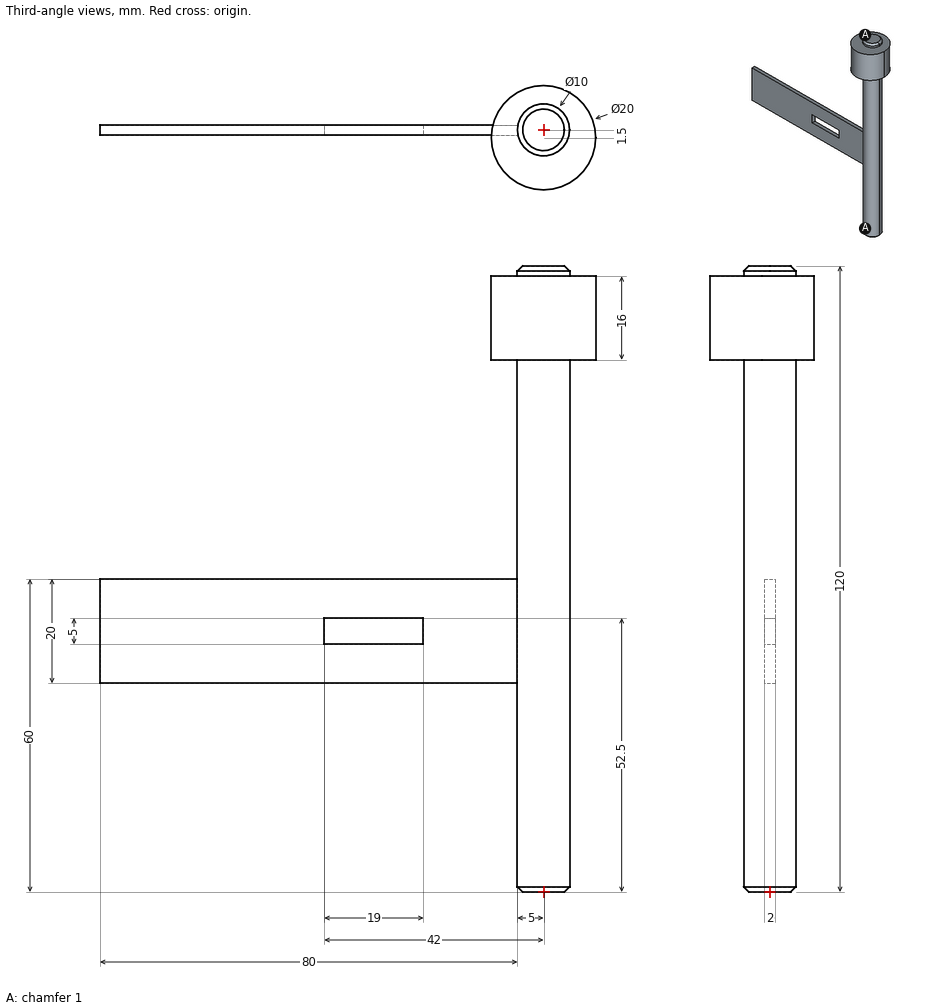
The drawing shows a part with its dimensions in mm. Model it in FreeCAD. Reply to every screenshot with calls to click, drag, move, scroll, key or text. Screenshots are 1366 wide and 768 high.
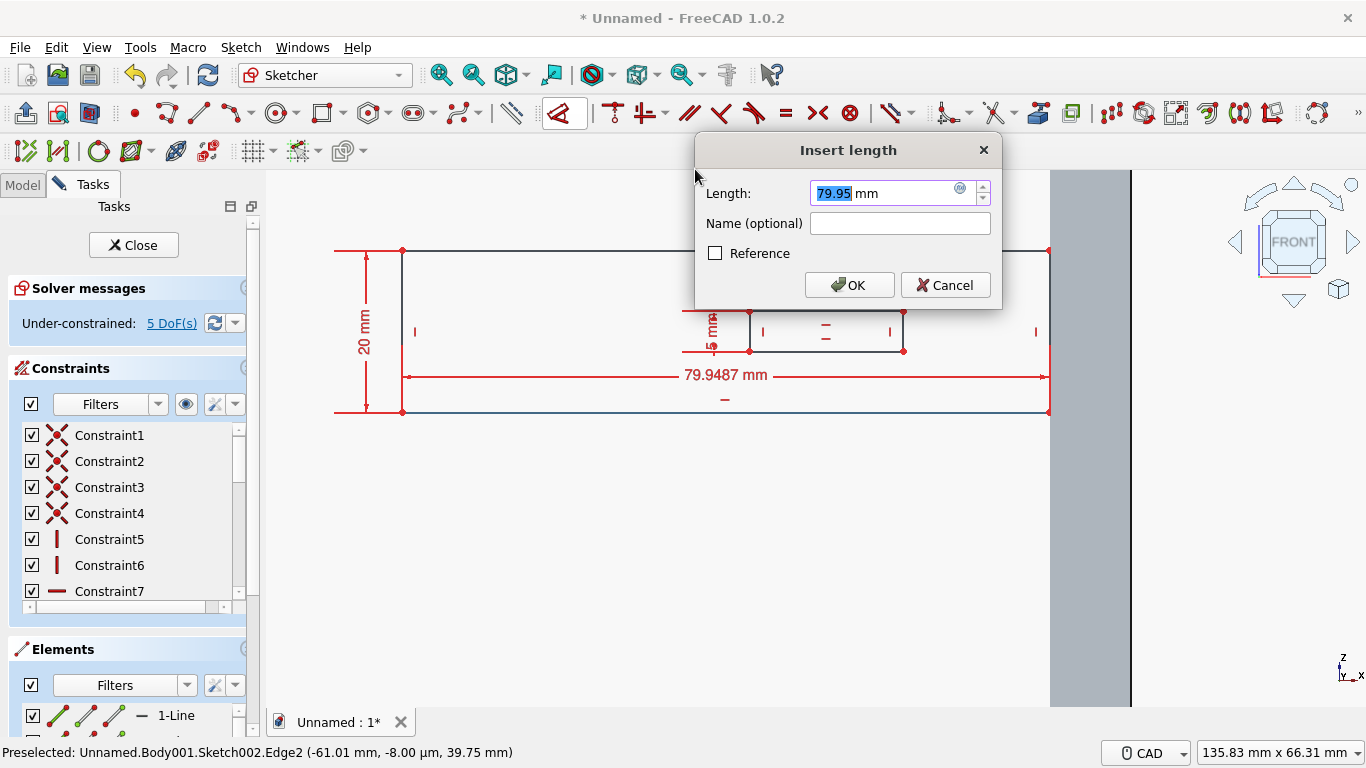
text(80)
key(Return)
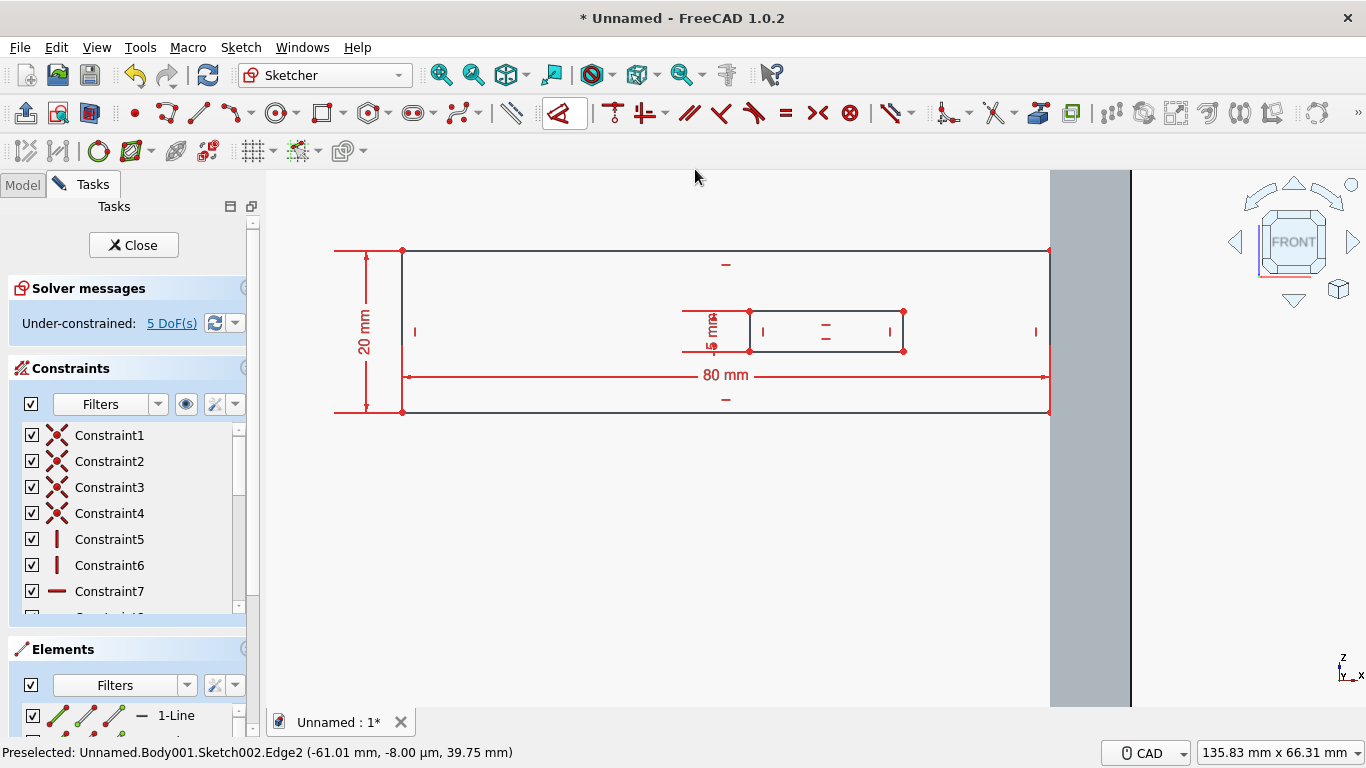
click(796, 352)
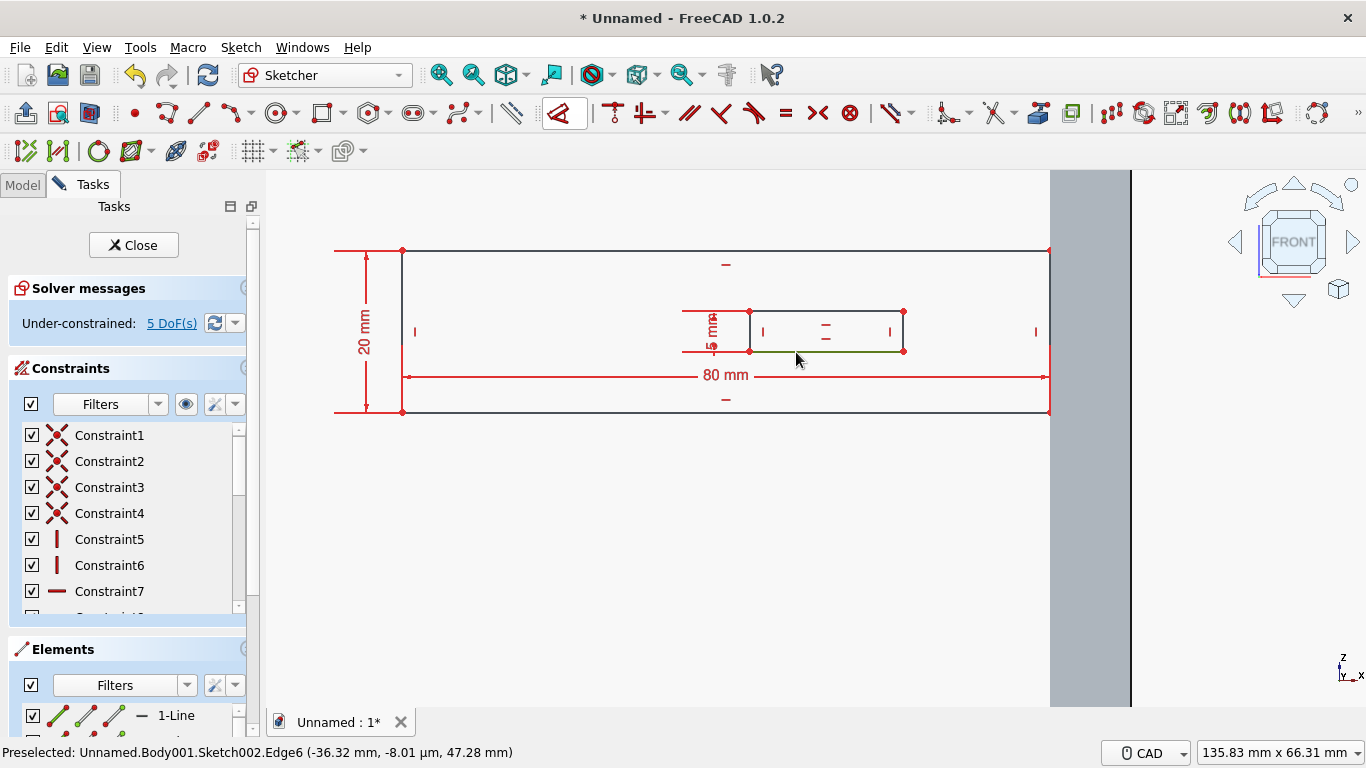
click(582, 114)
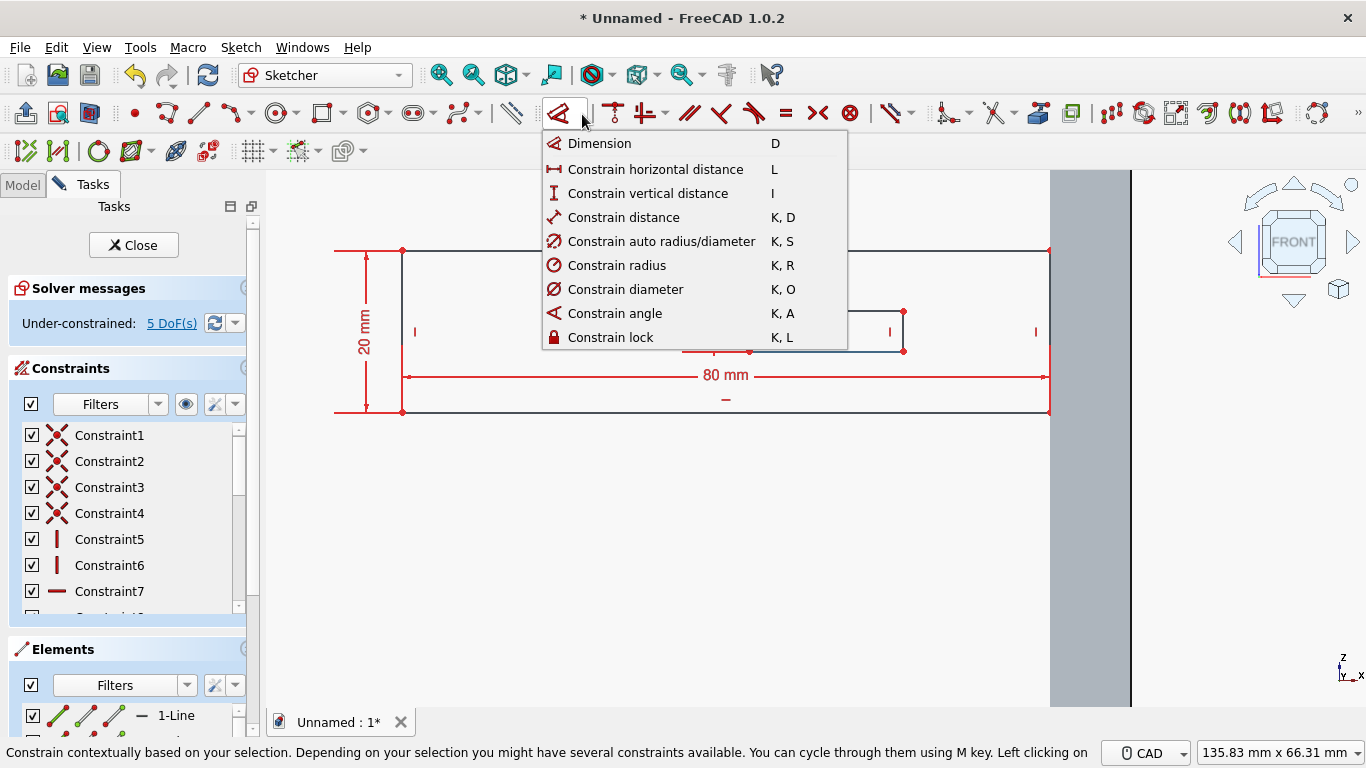
click(695, 169)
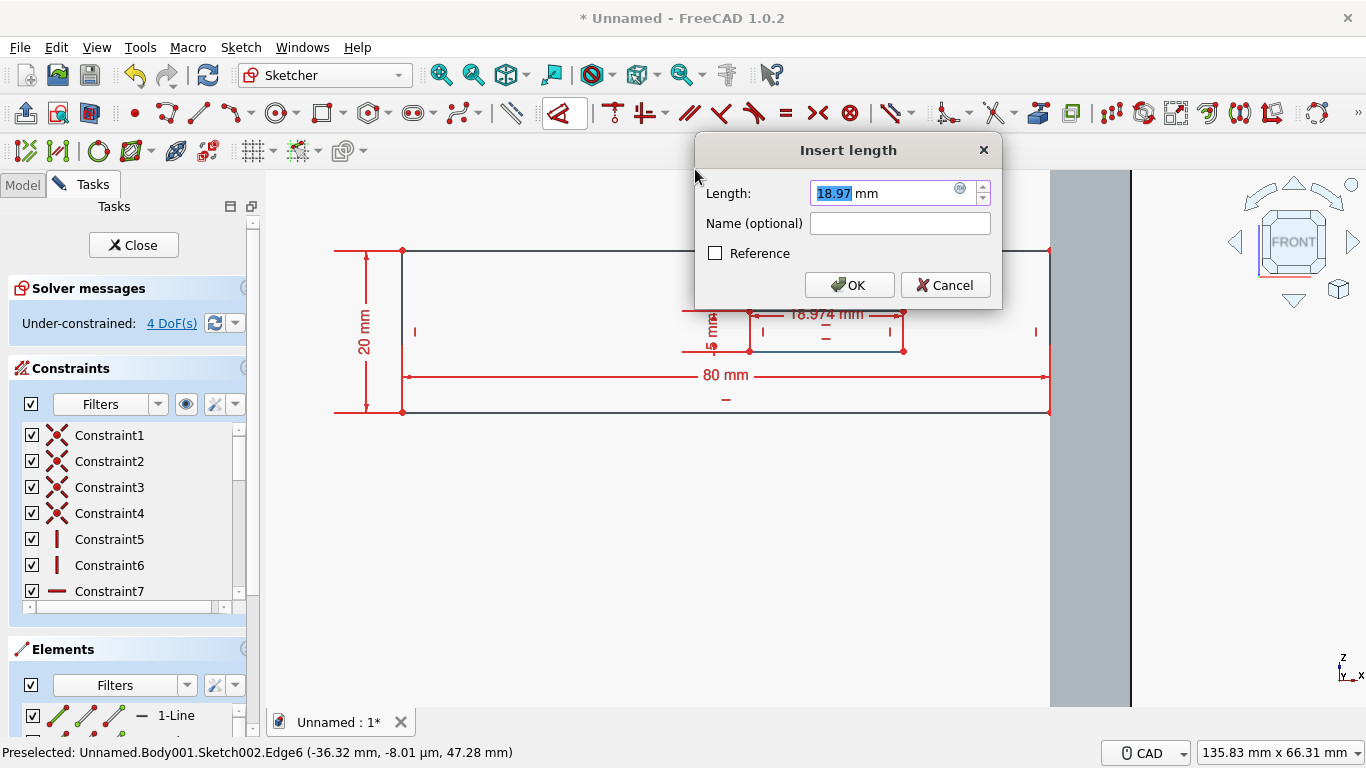
text(19)
key(Return)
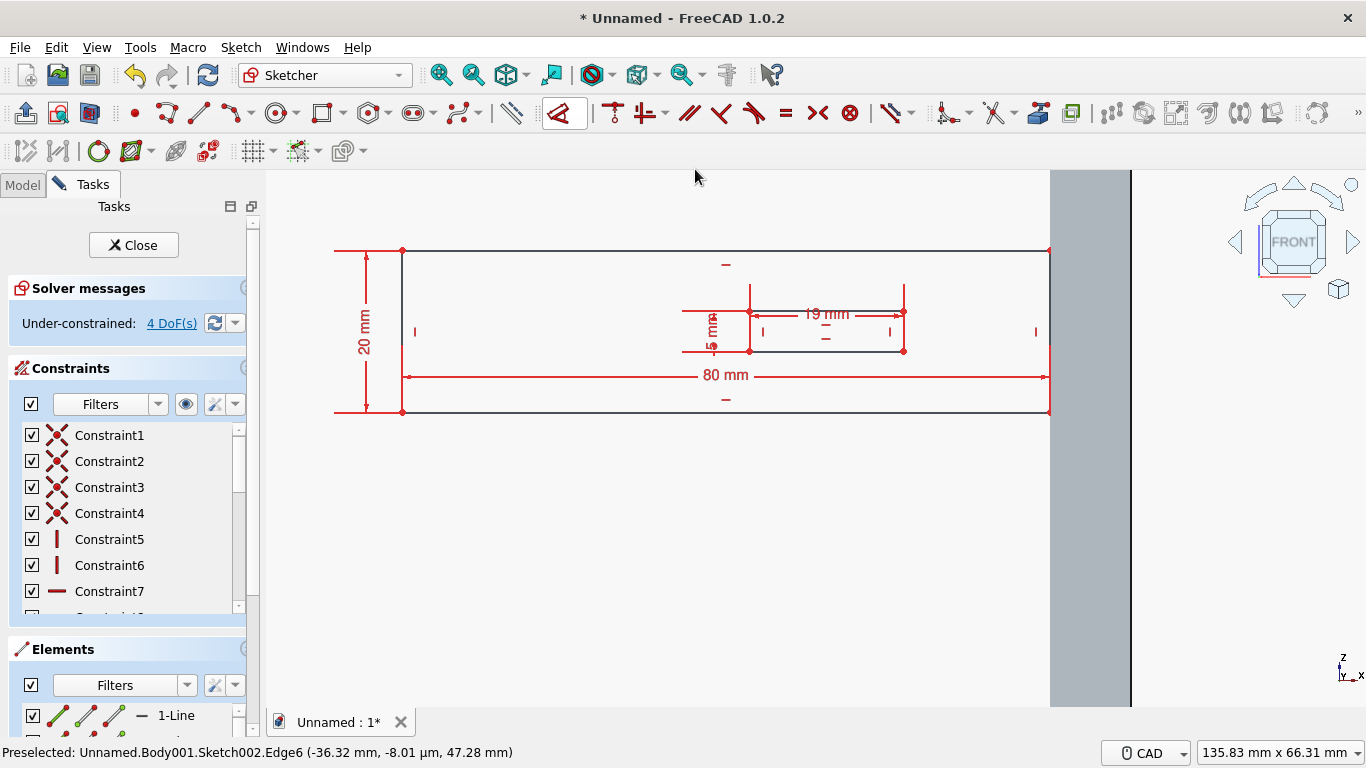
click(1050, 413)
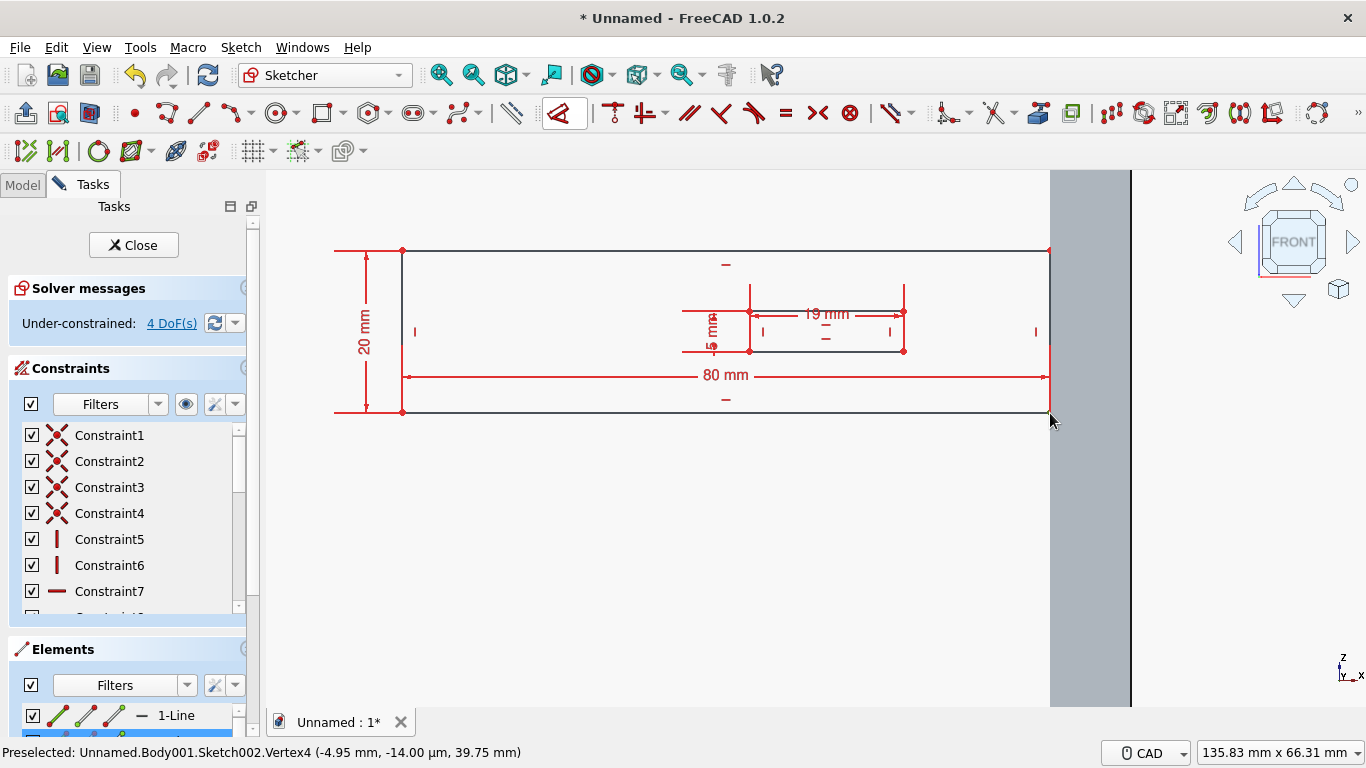
click(582, 114)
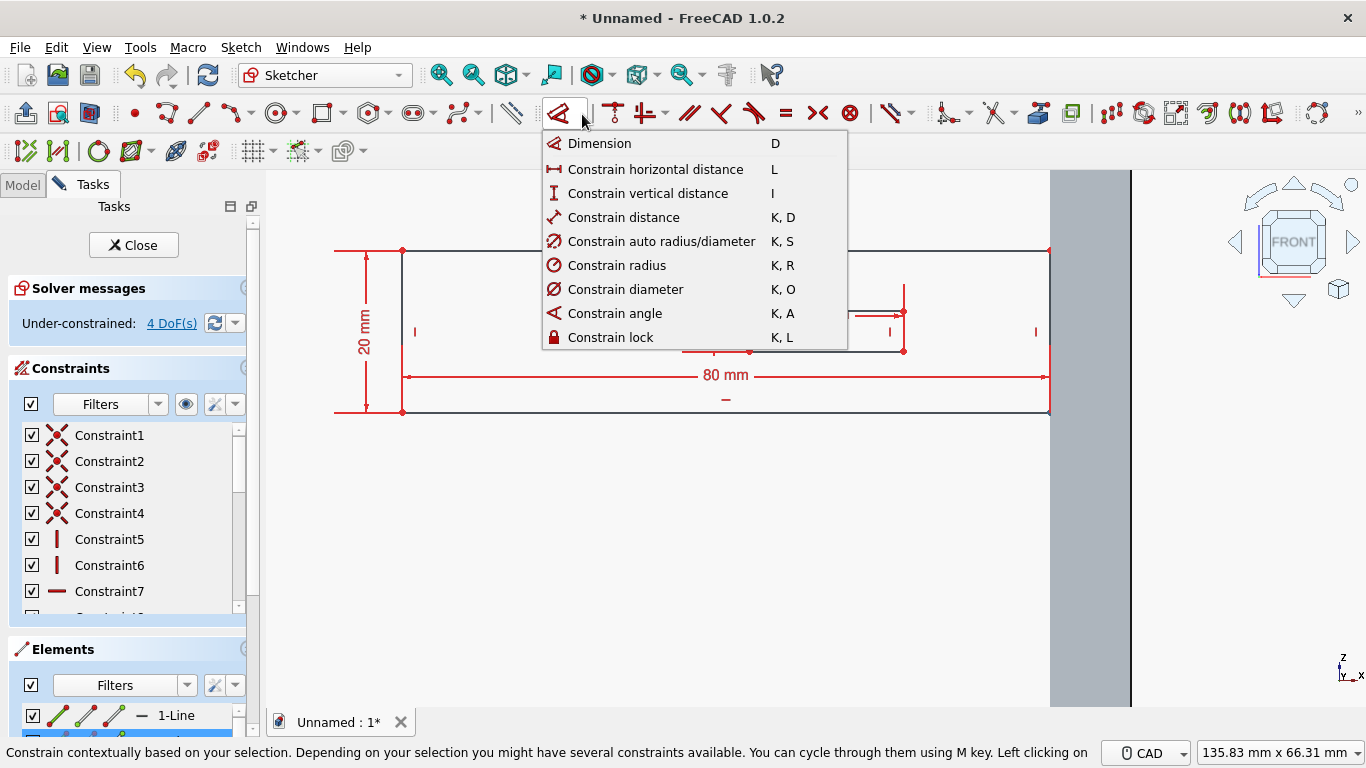
click(695, 169)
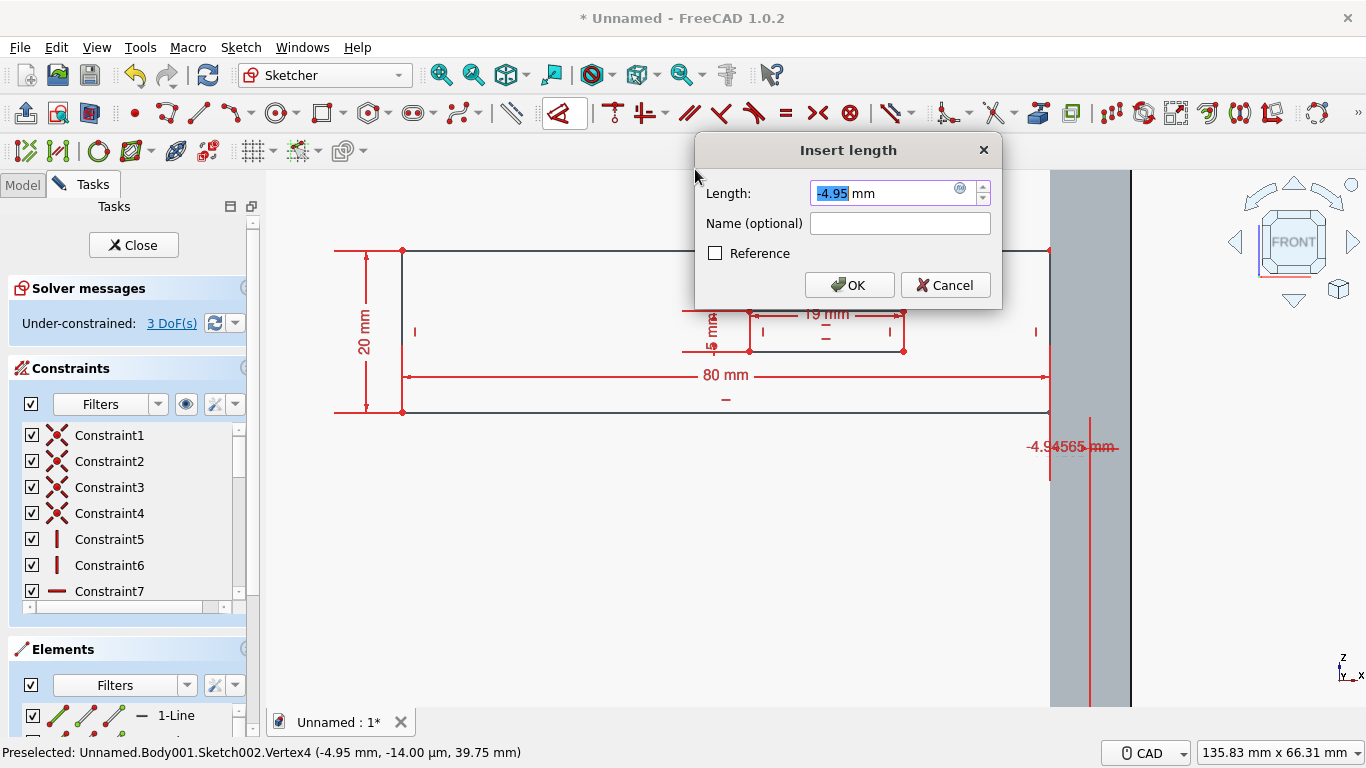
text(-5)
key(Return)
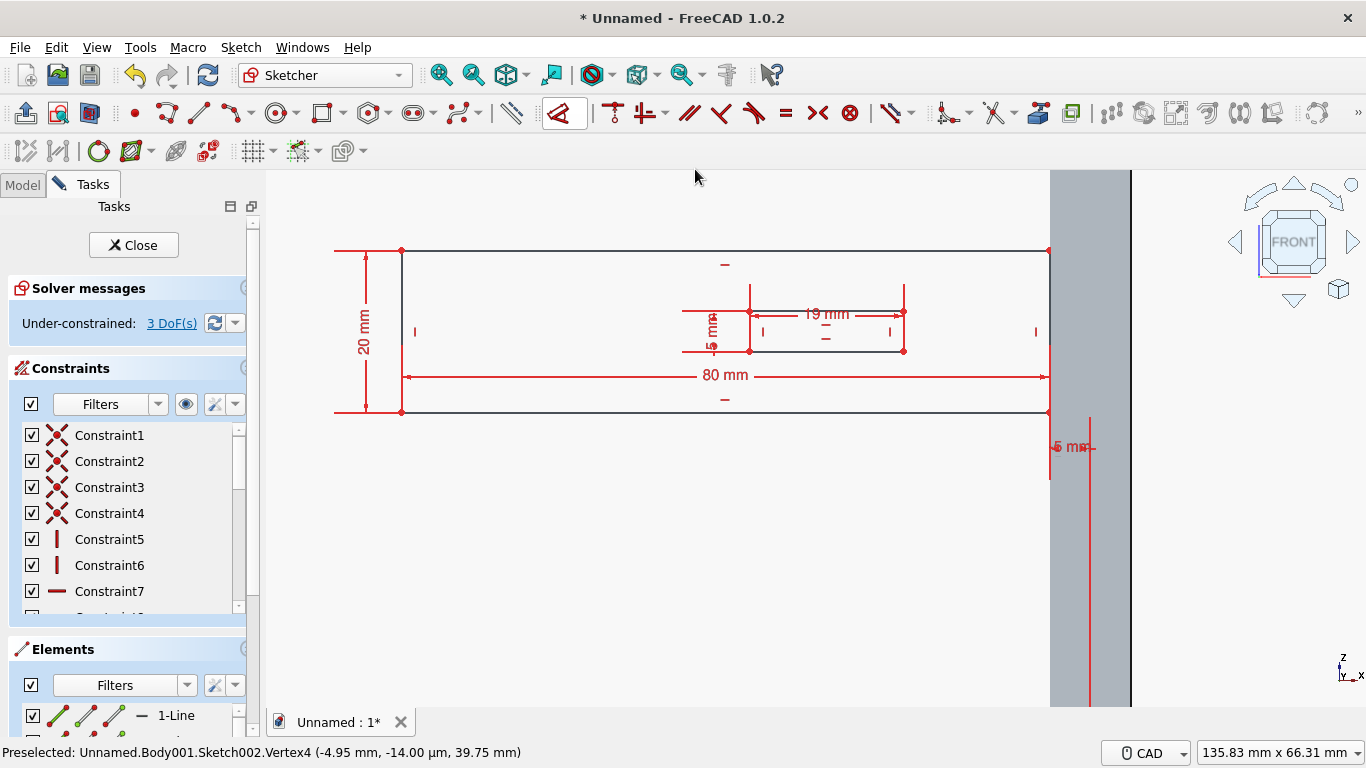
click(402, 251)